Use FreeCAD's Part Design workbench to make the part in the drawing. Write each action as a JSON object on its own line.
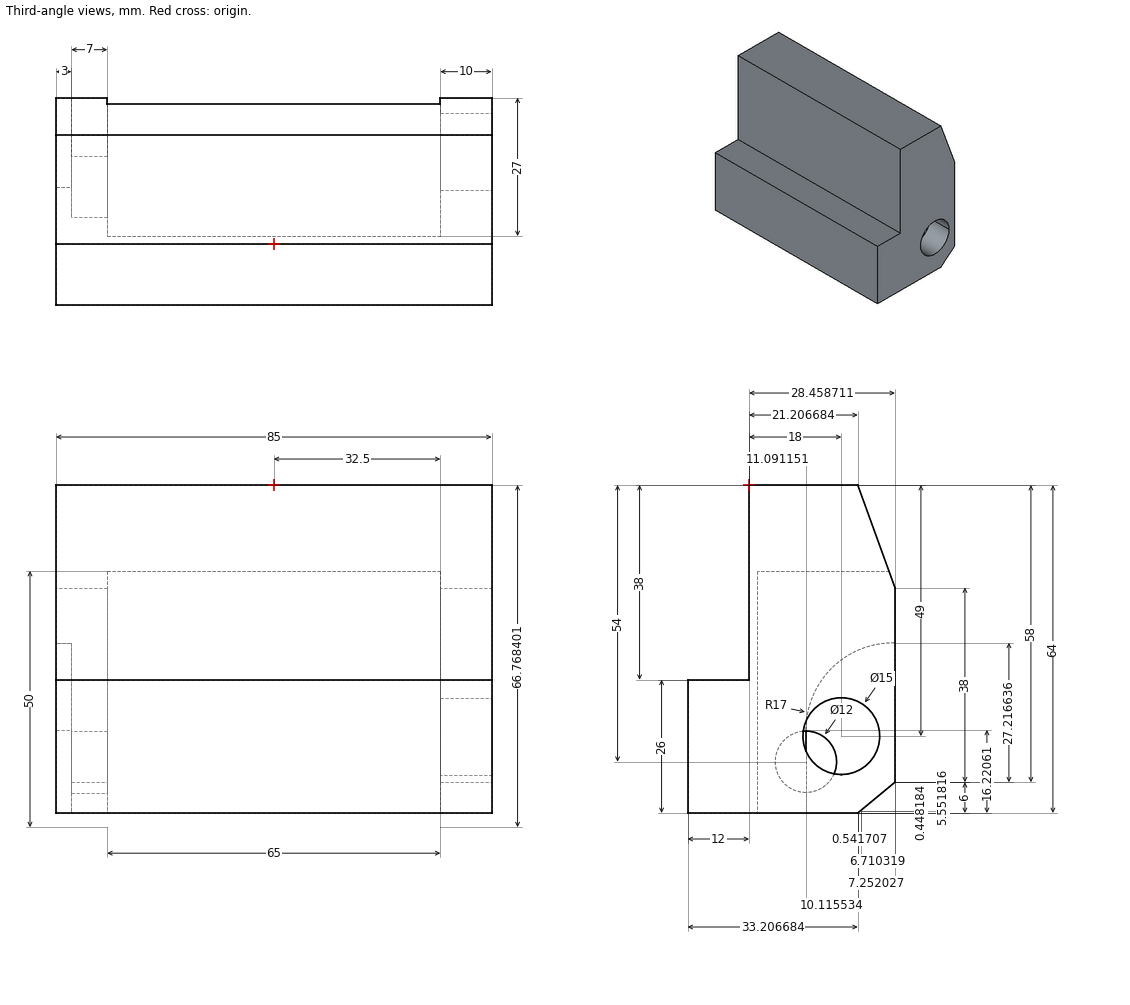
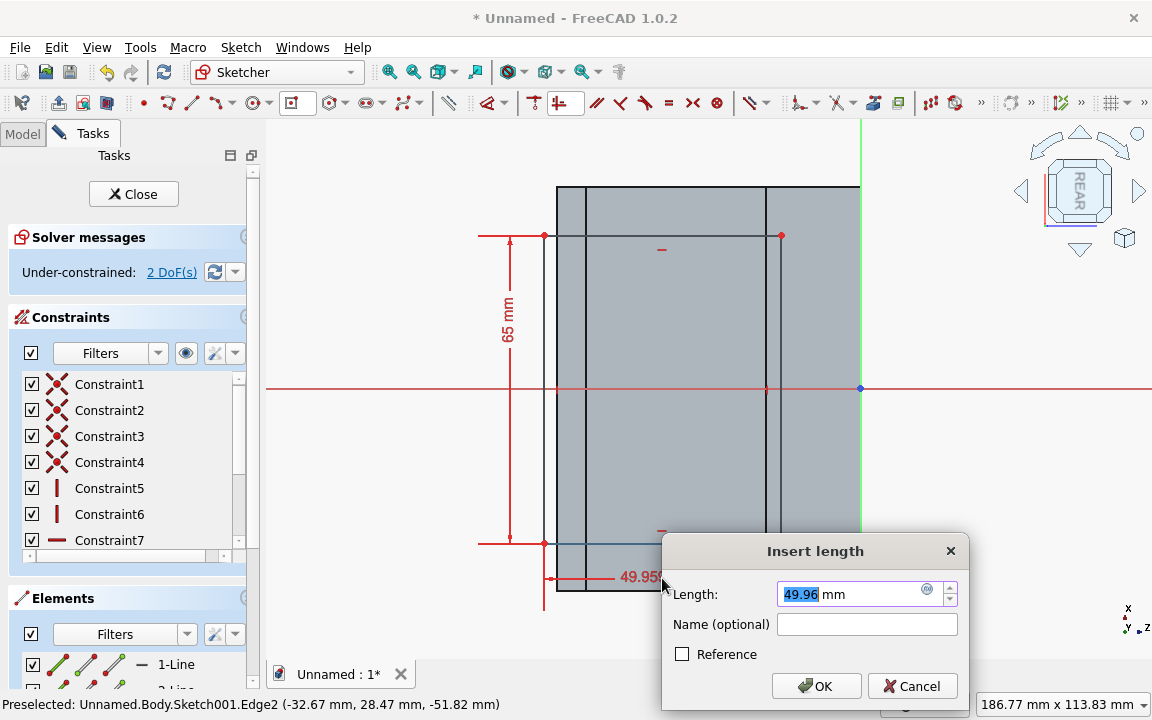
{"action": "type", "text": "50"}
{"action": "key", "text": "Return"}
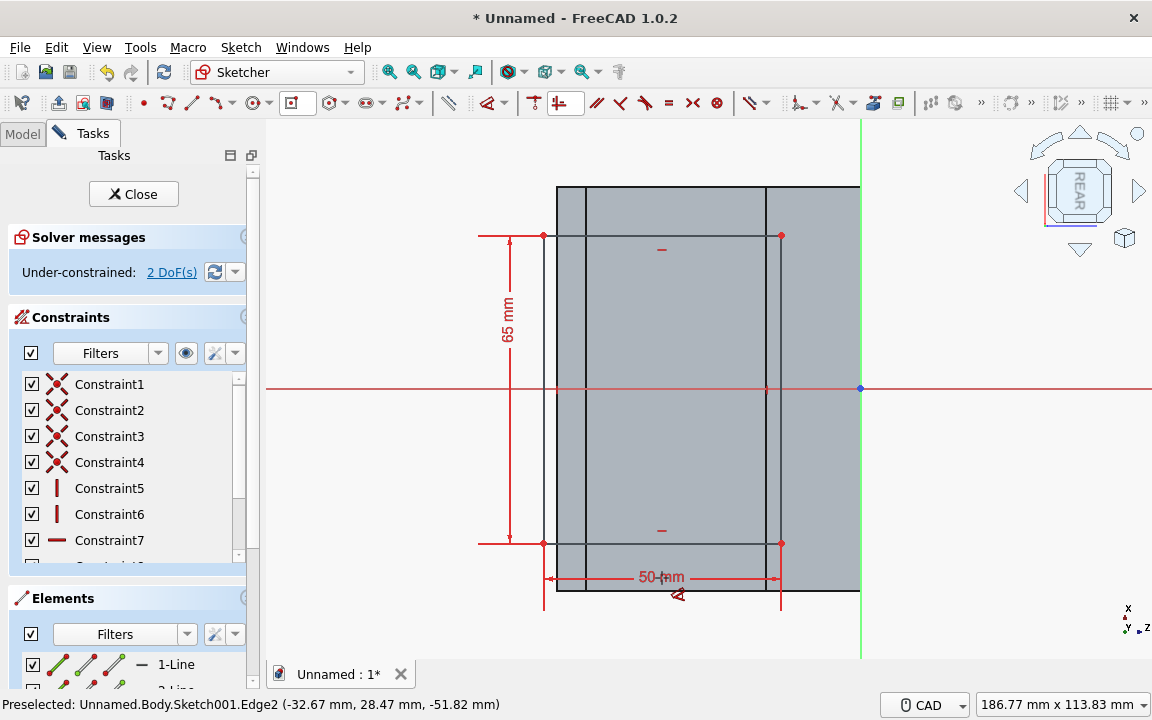
{"action": "left_click", "coordinate": [544, 236]}
{"action": "left_click", "coordinate": [510, 277]}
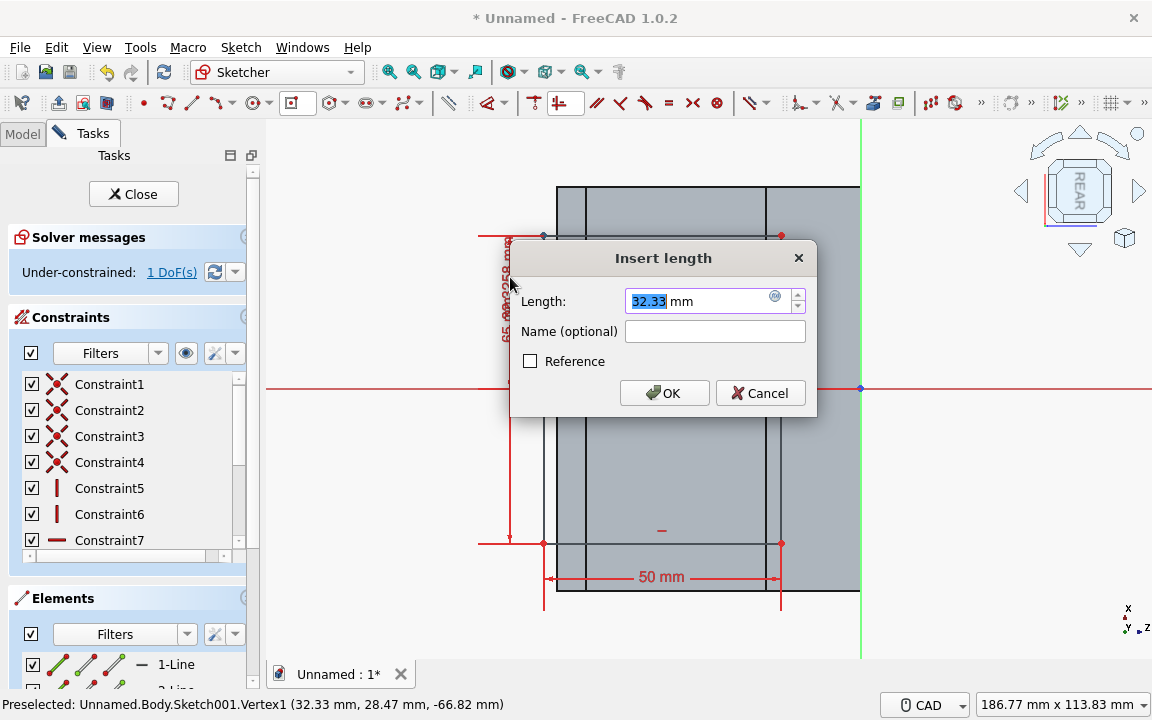
{"action": "type", "text": "32.5"}
{"action": "key", "text": "Return"}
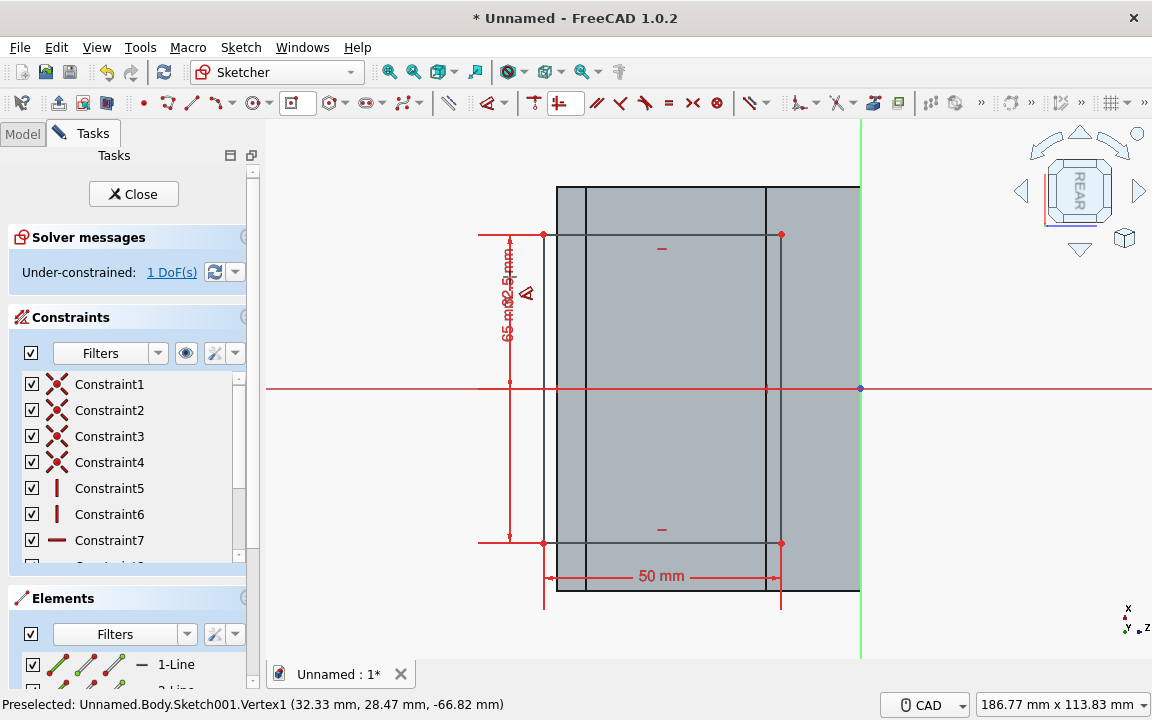
{"action": "left_click", "coordinate": [544, 235]}
{"action": "left_click", "coordinate": [702, 201]}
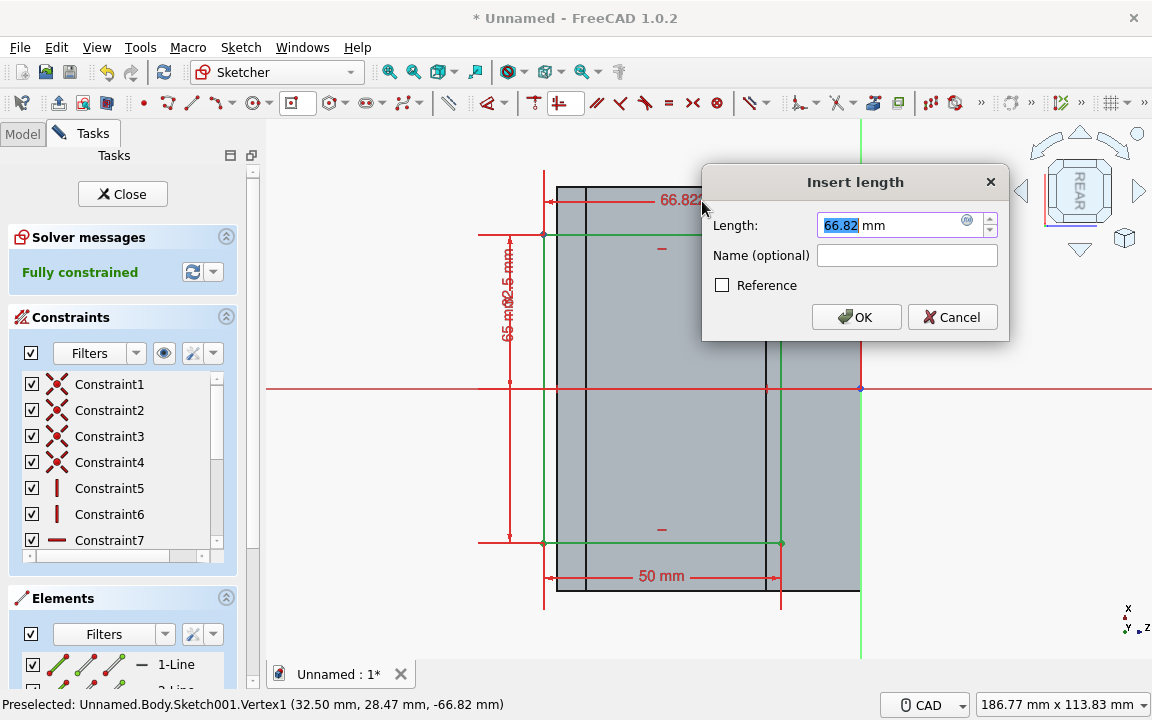
{"action": "type", "text": "66.768401"}
{"action": "key", "text": "Return"}
{"action": "key", "text": "Escape"}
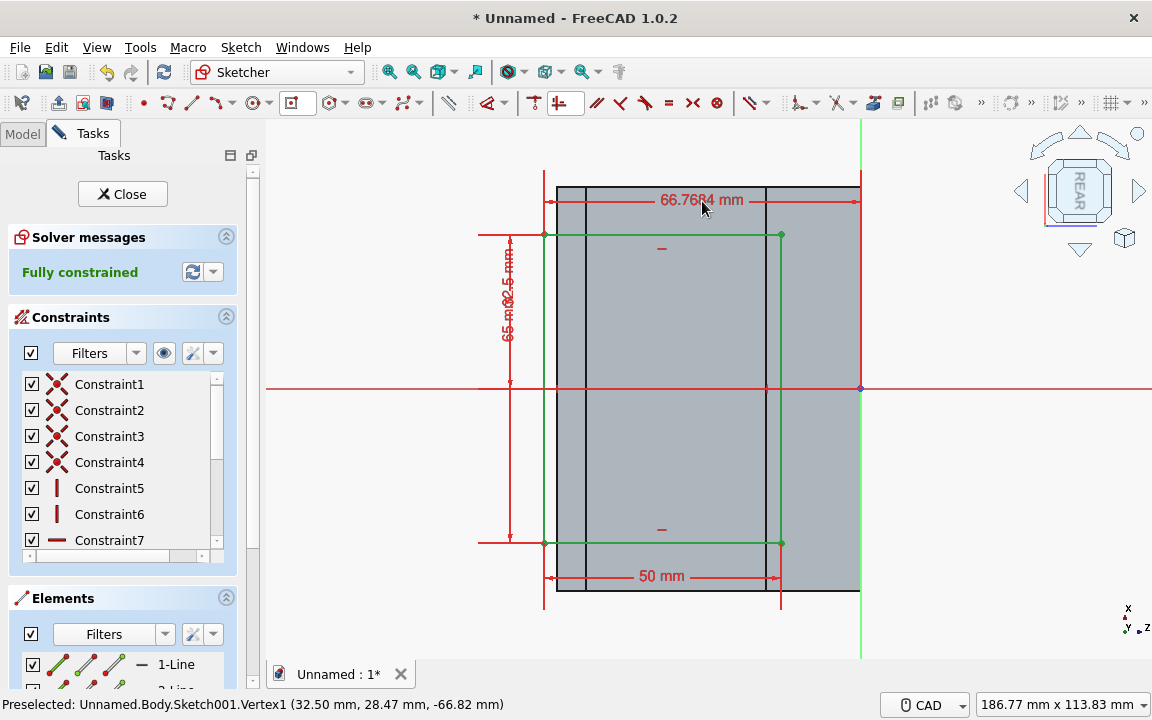
{"action": "left_click", "coordinate": [123, 194]}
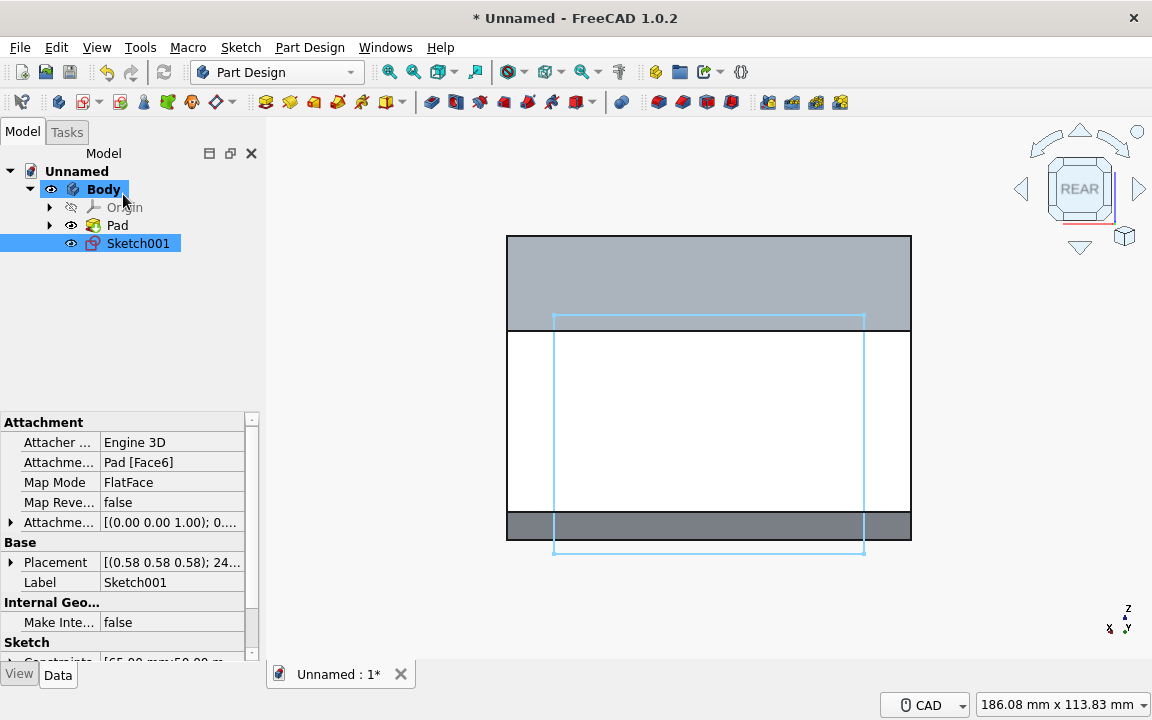
{"action": "left_click", "coordinate": [432, 102]}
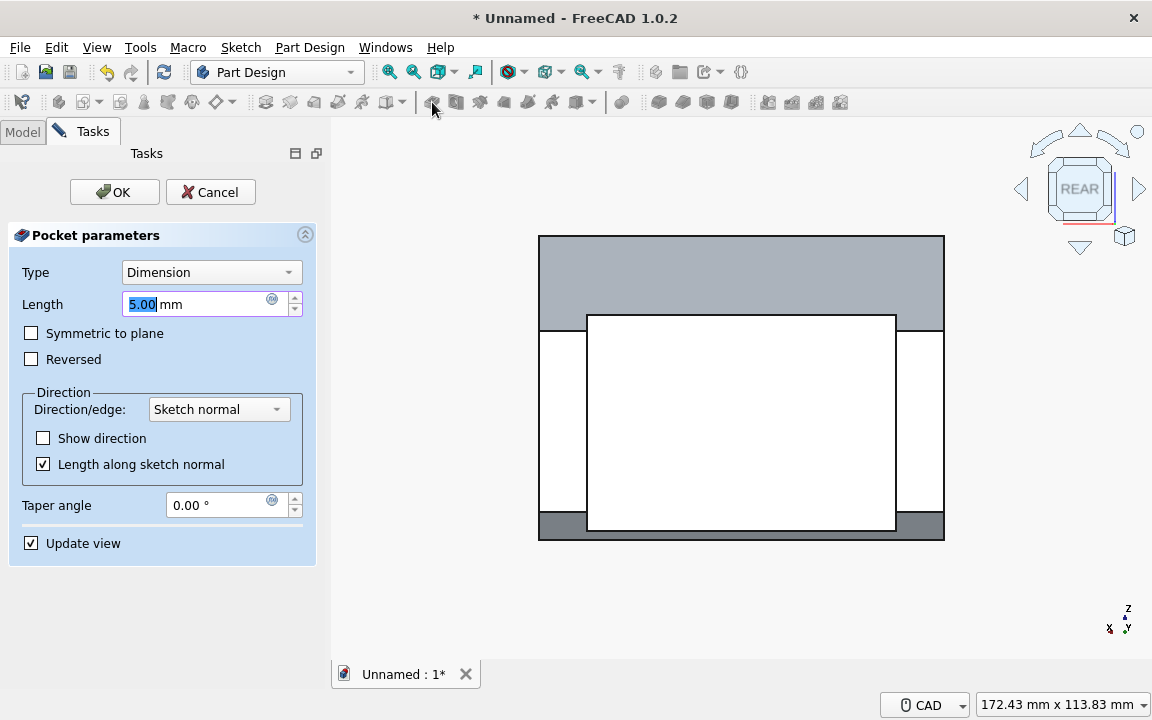
{"action": "type", "text": "27"}
{"action": "key", "text": "Tab"}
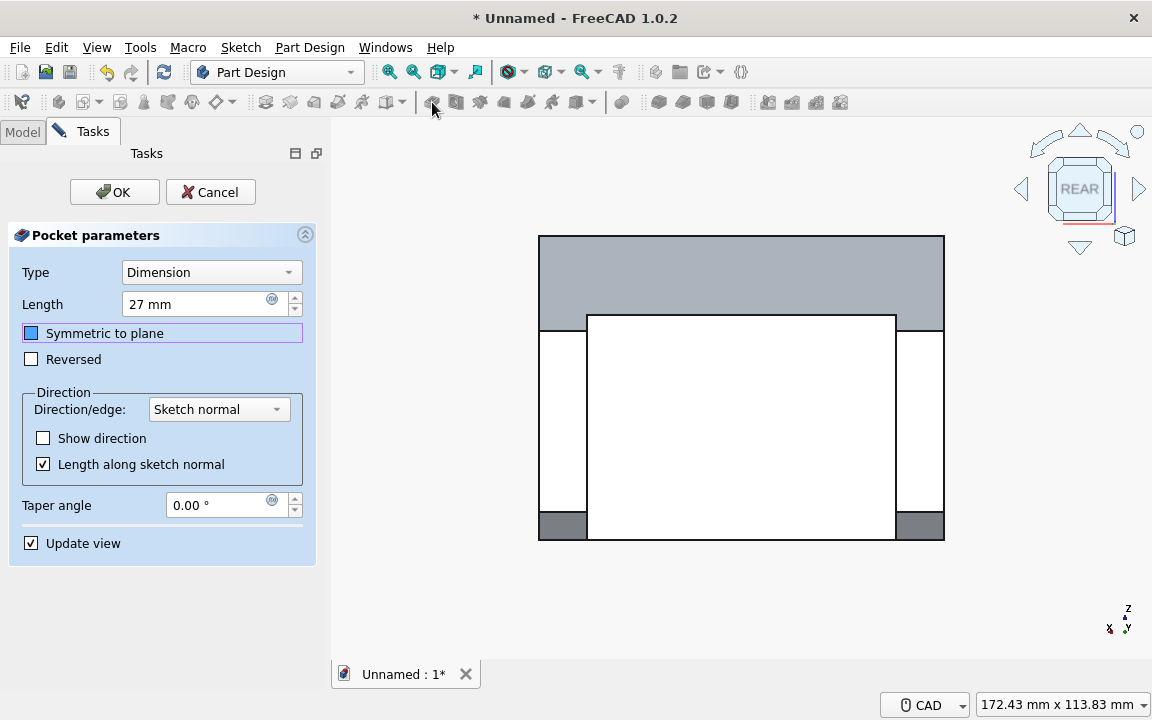
{"action": "left_click", "coordinate": [115, 192]}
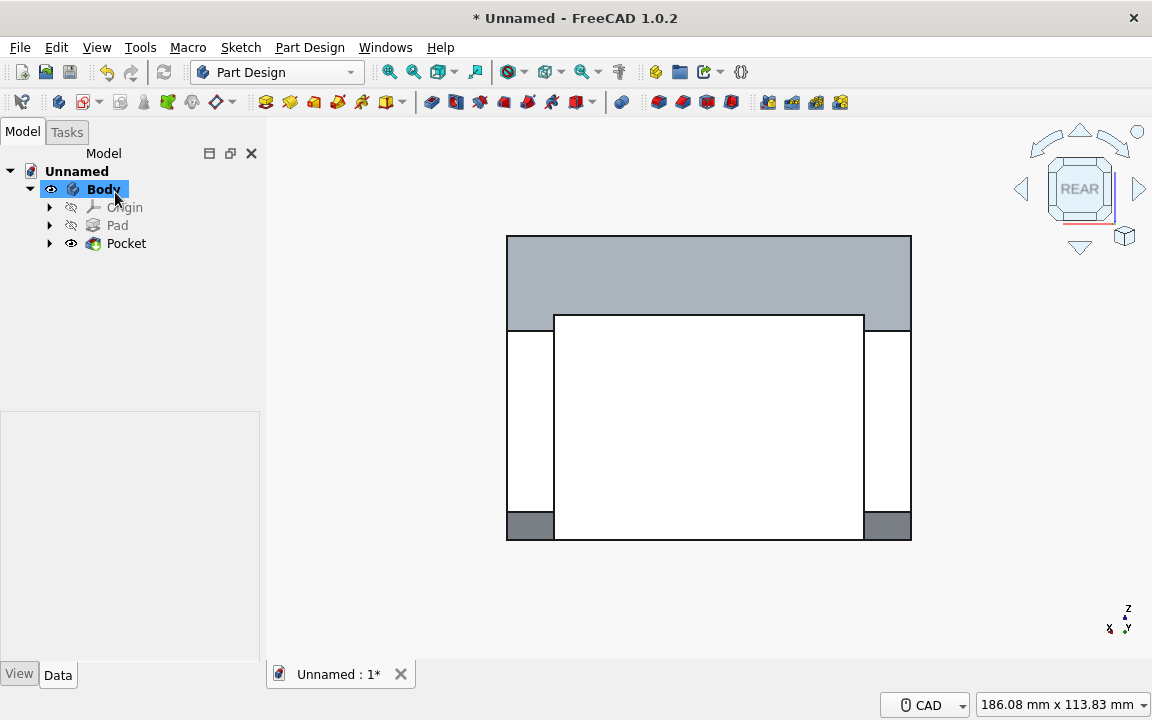
{"action": "key", "text": "0"}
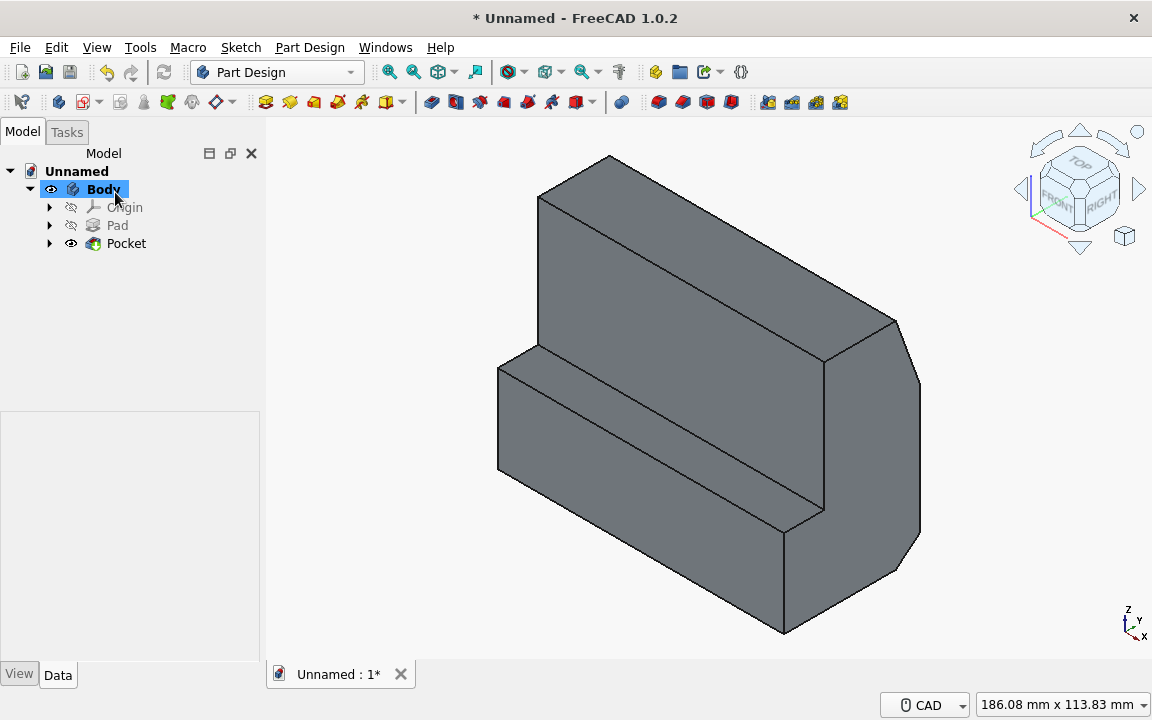
{"action": "left_click", "coordinate": [872, 494]}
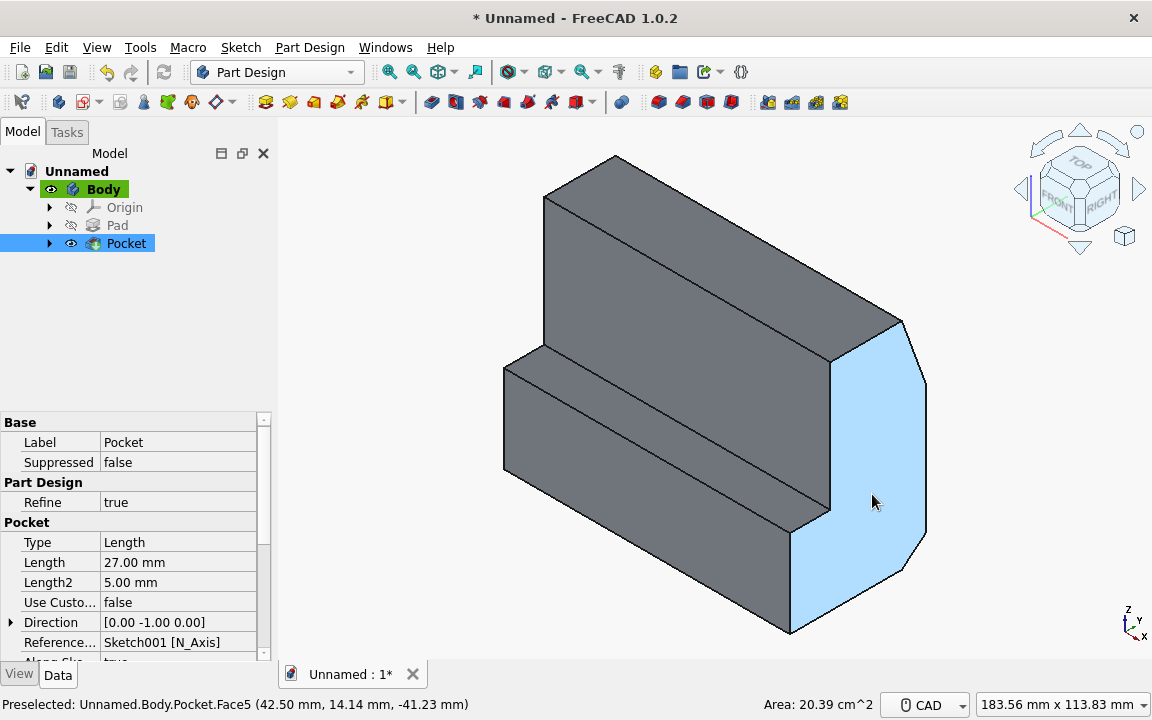
{"action": "left_click", "coordinate": [84, 102]}